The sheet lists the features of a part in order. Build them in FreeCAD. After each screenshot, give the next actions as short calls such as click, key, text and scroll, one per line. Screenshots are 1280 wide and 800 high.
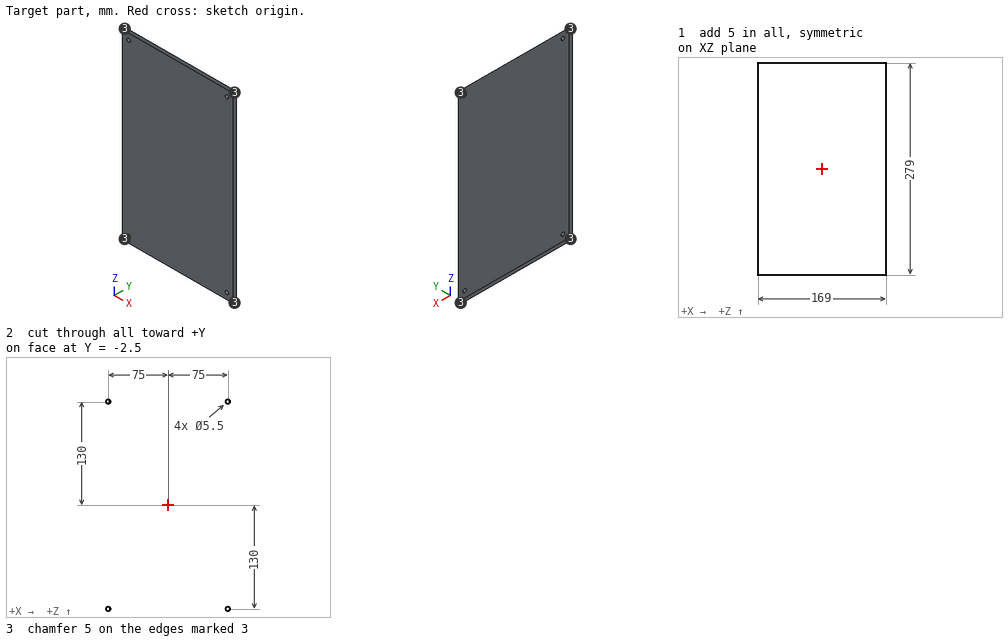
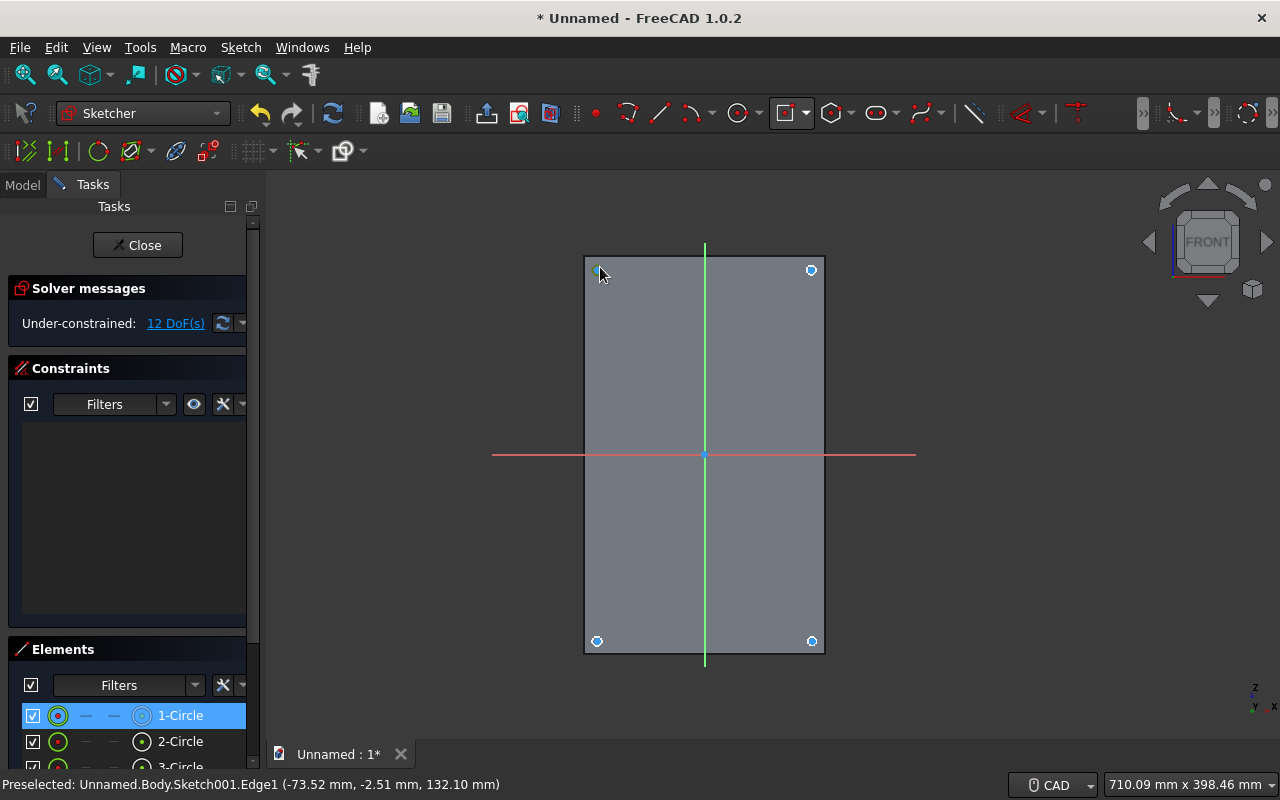
scroll(815, 267, up, 6)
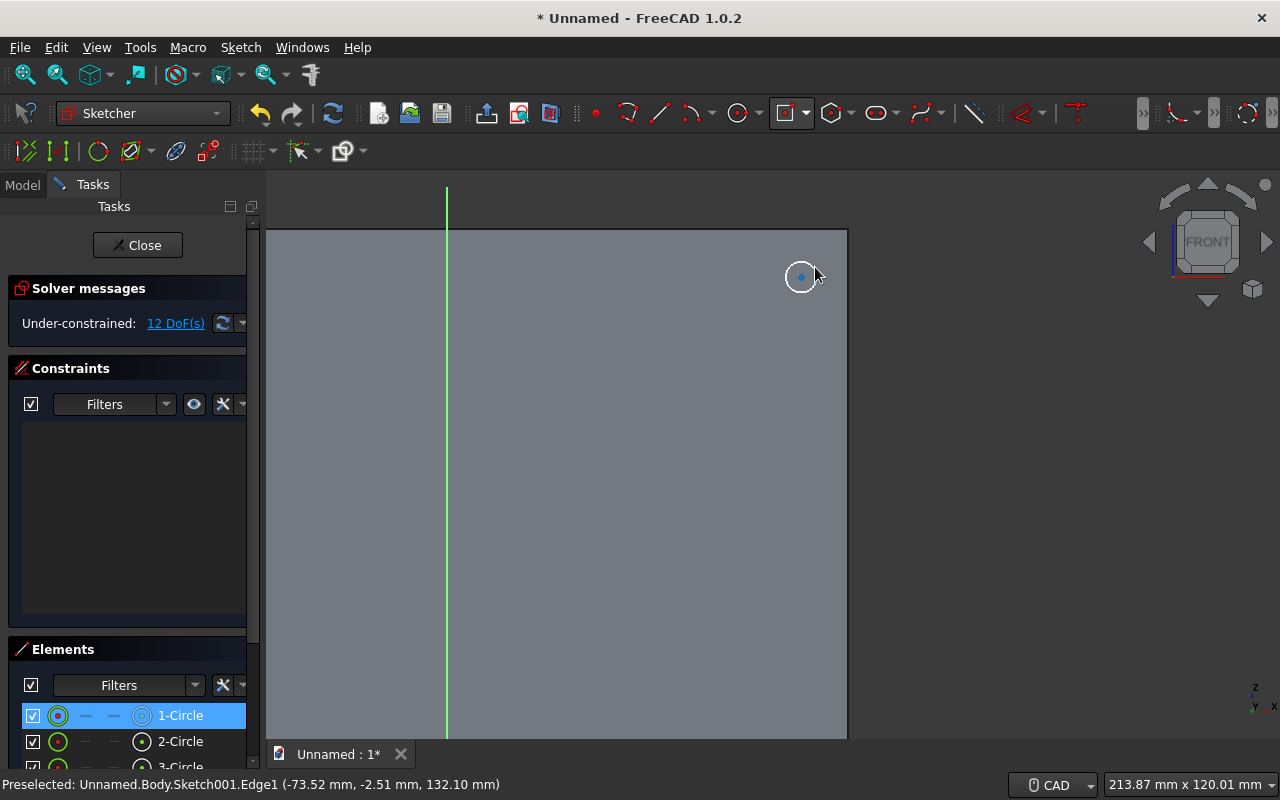
click(812, 266)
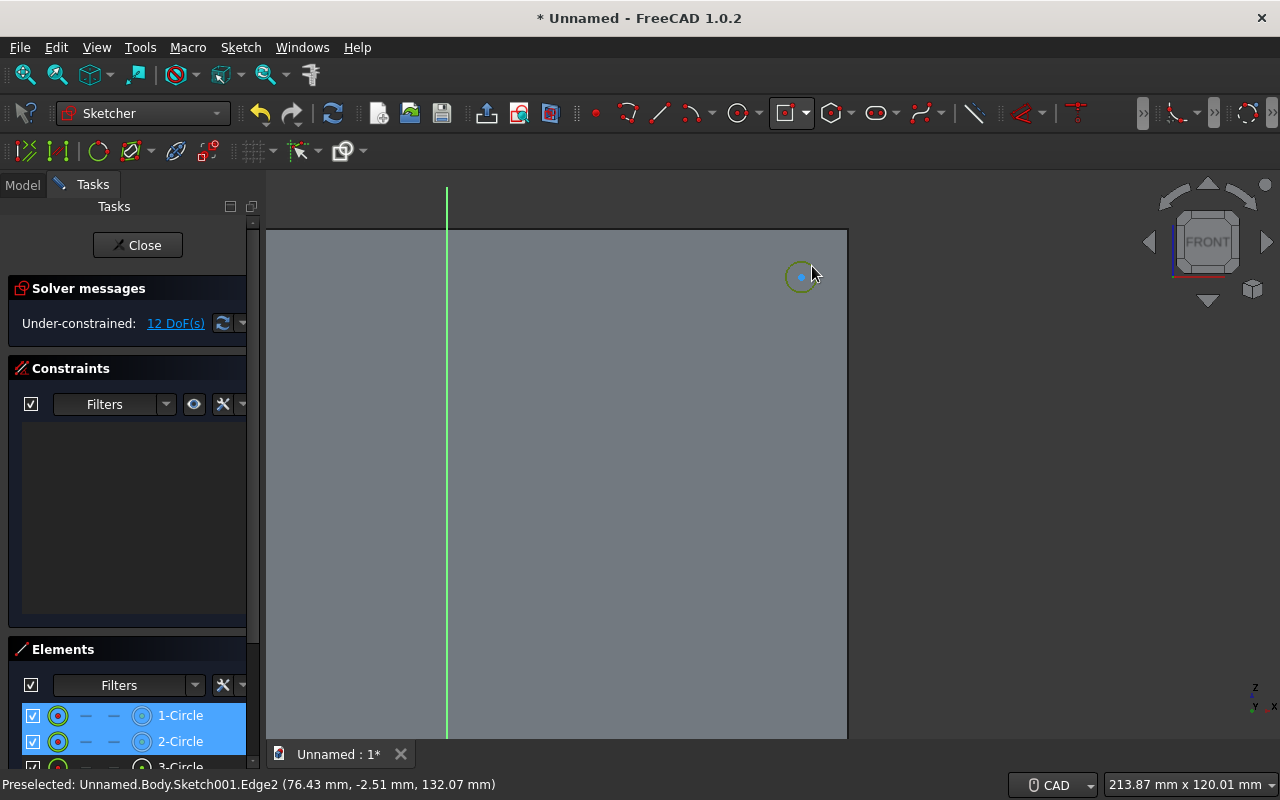
scroll(815, 267, down, 6)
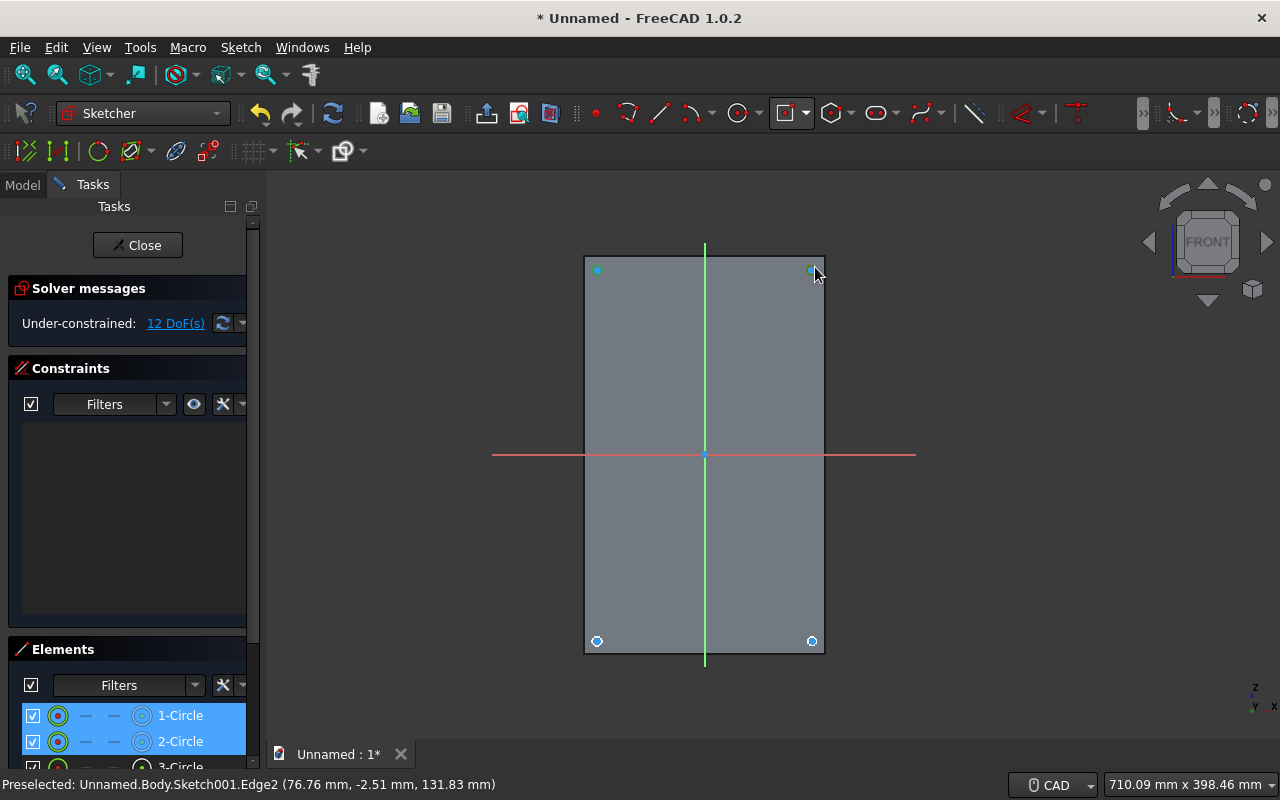
scroll(815, 638, up, 7)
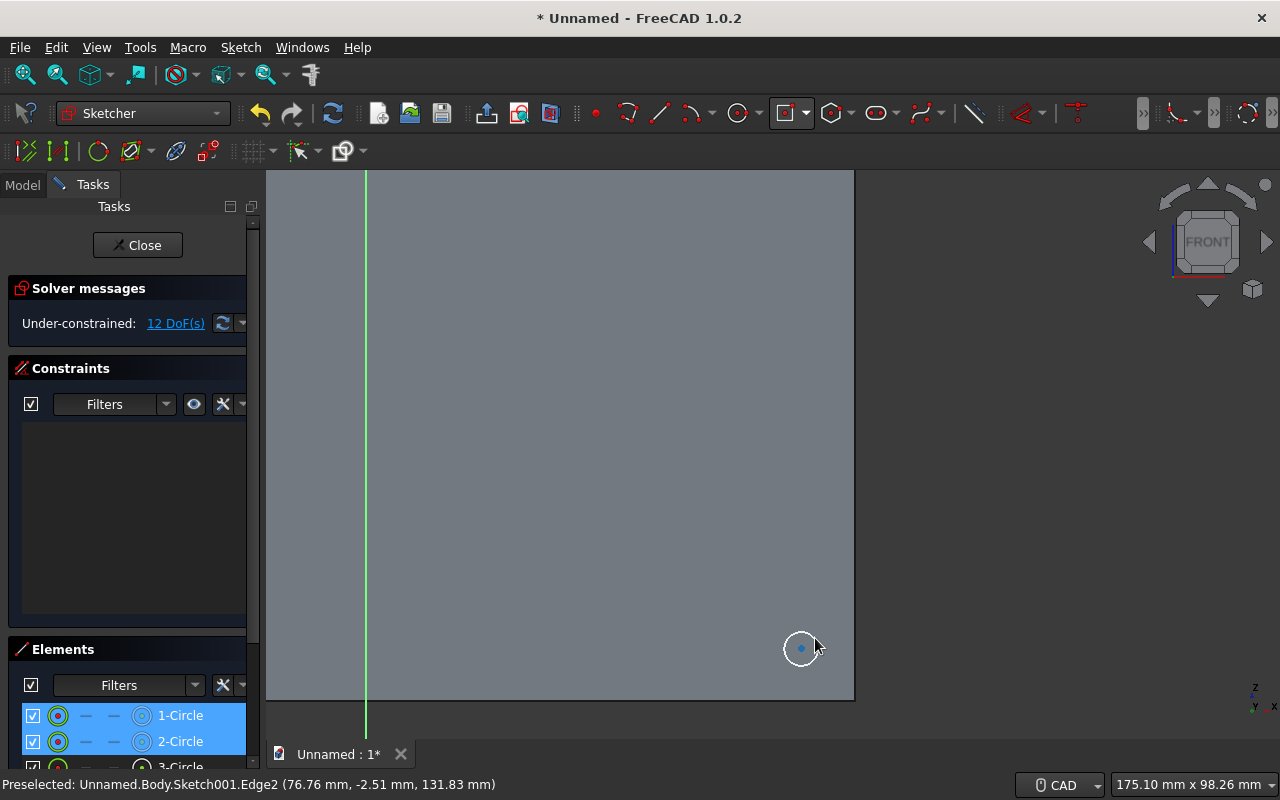
click(813, 637)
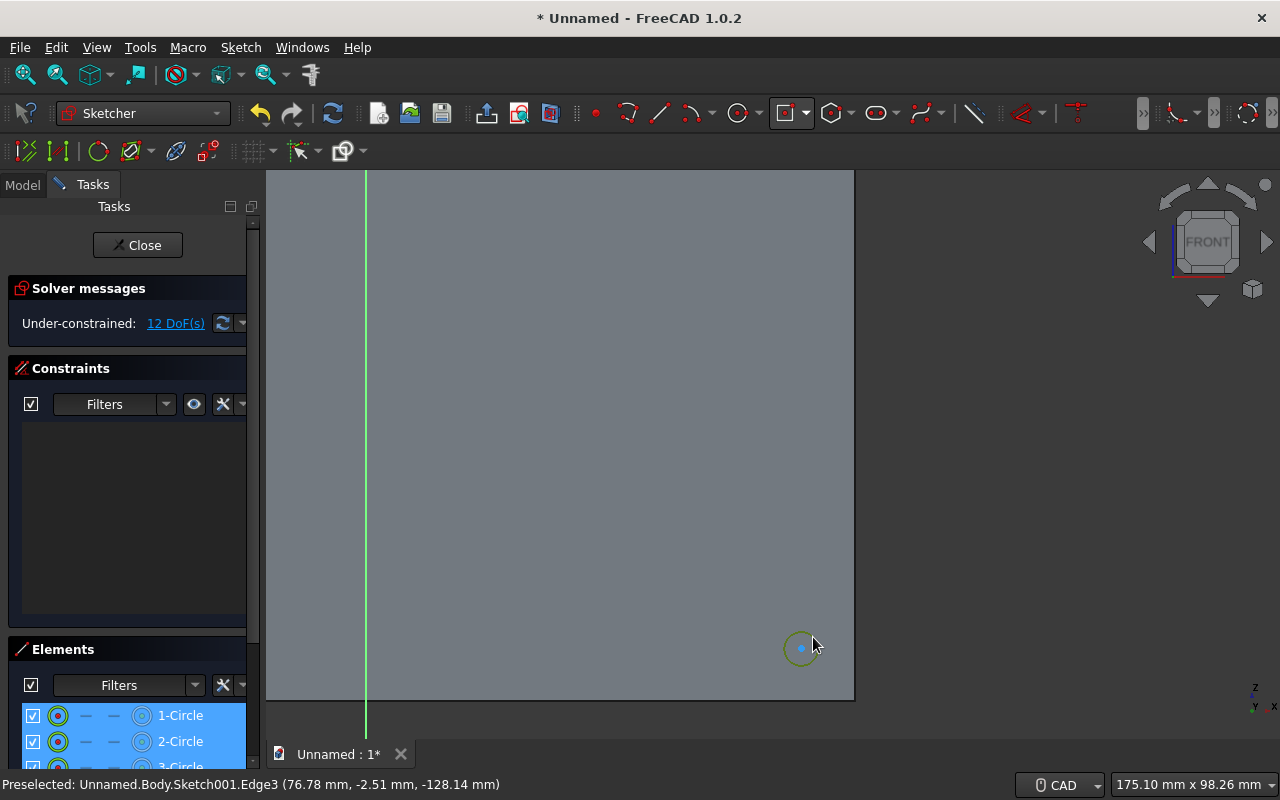
scroll(815, 638, down, 7)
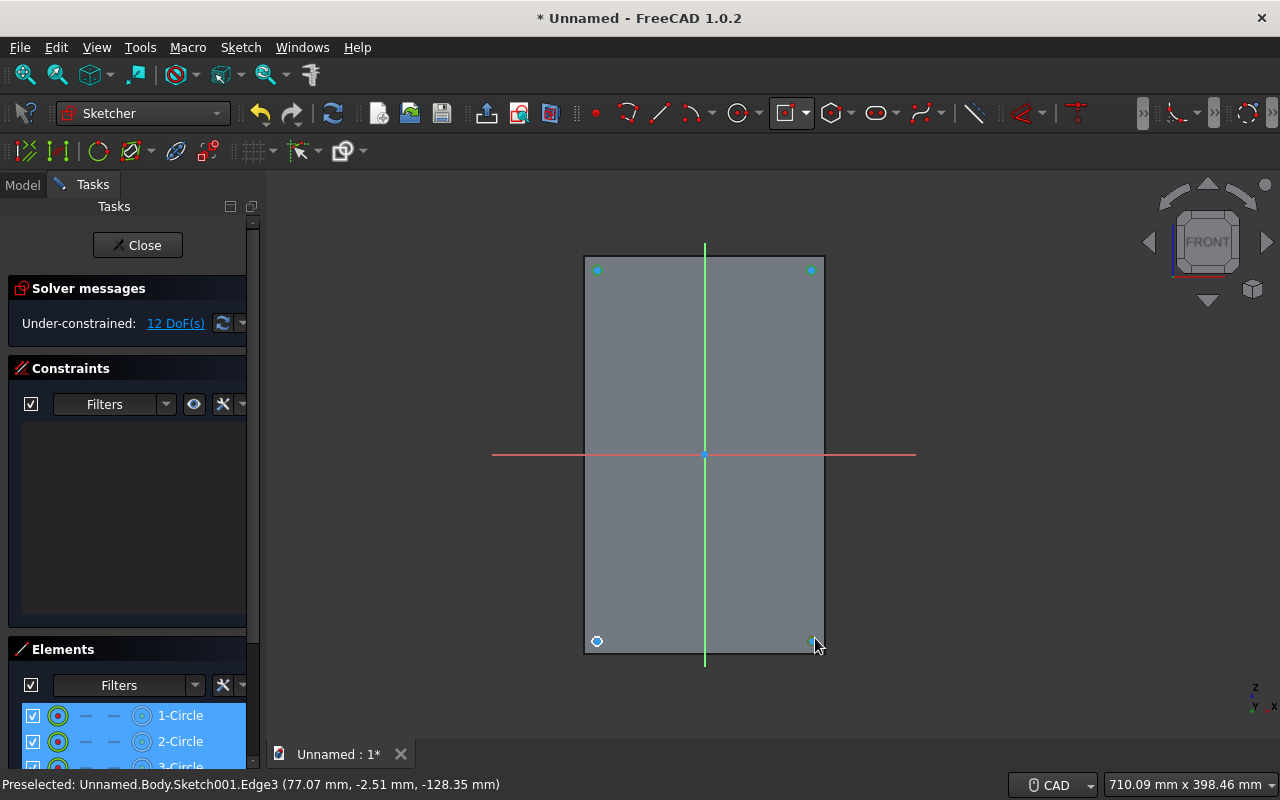
scroll(600, 638, up, 6)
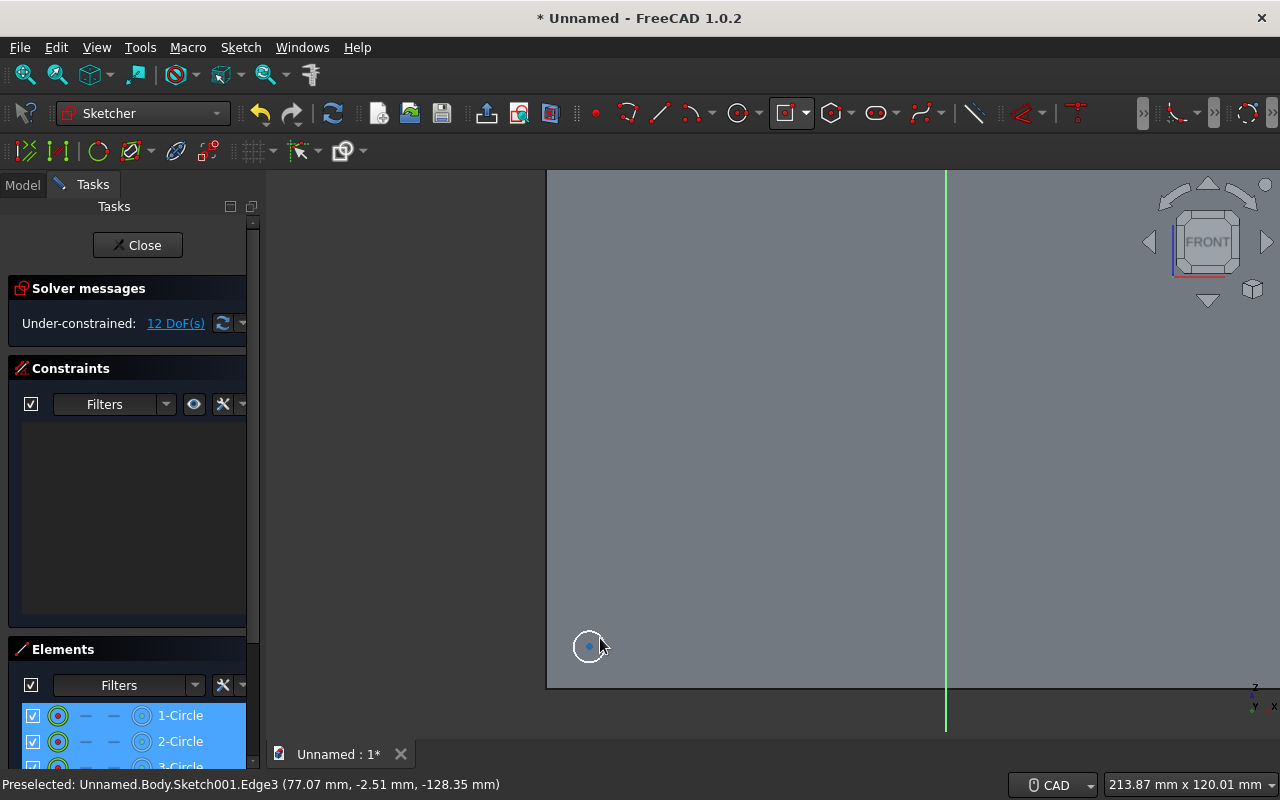
click(600, 636)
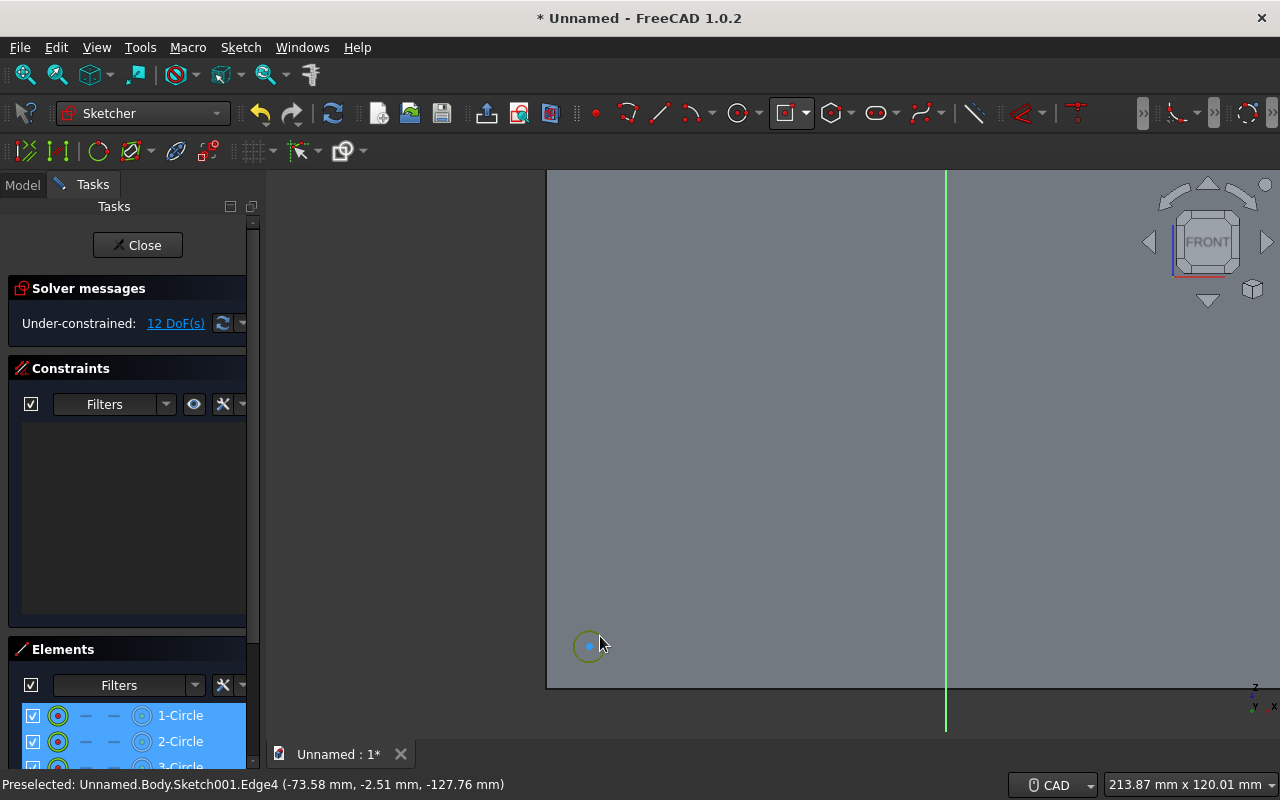
key(e)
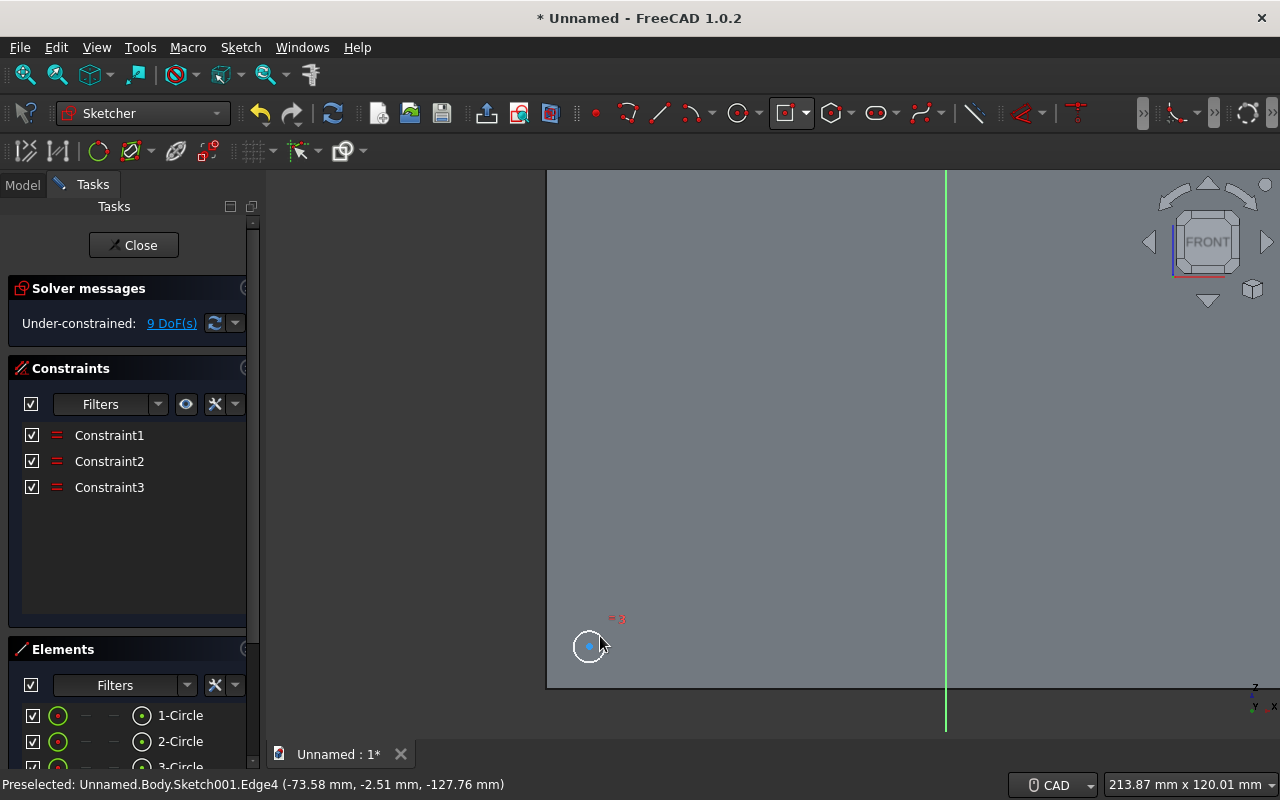
scroll(600, 638, down, 6)